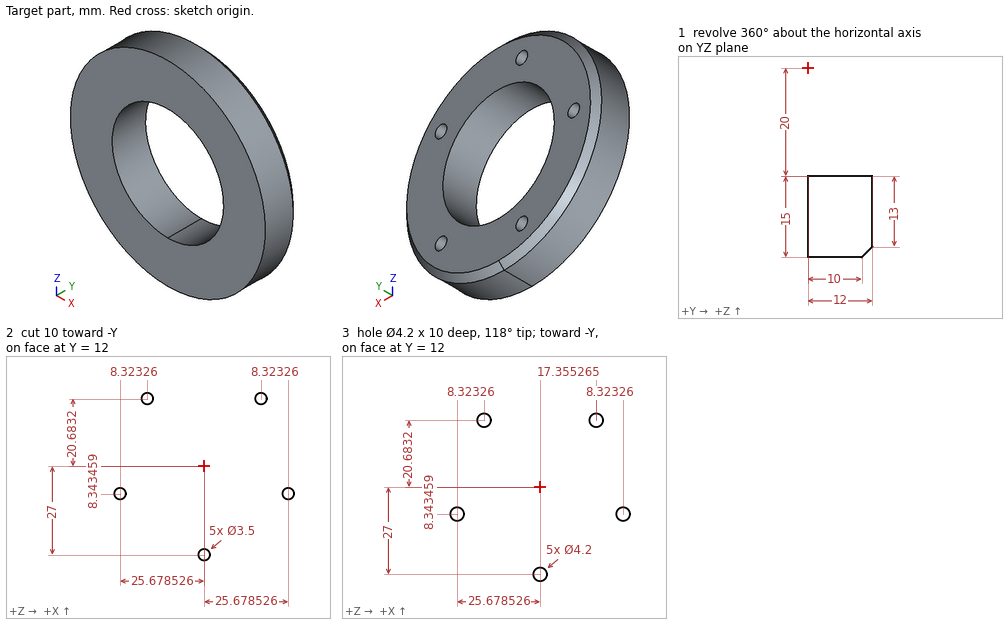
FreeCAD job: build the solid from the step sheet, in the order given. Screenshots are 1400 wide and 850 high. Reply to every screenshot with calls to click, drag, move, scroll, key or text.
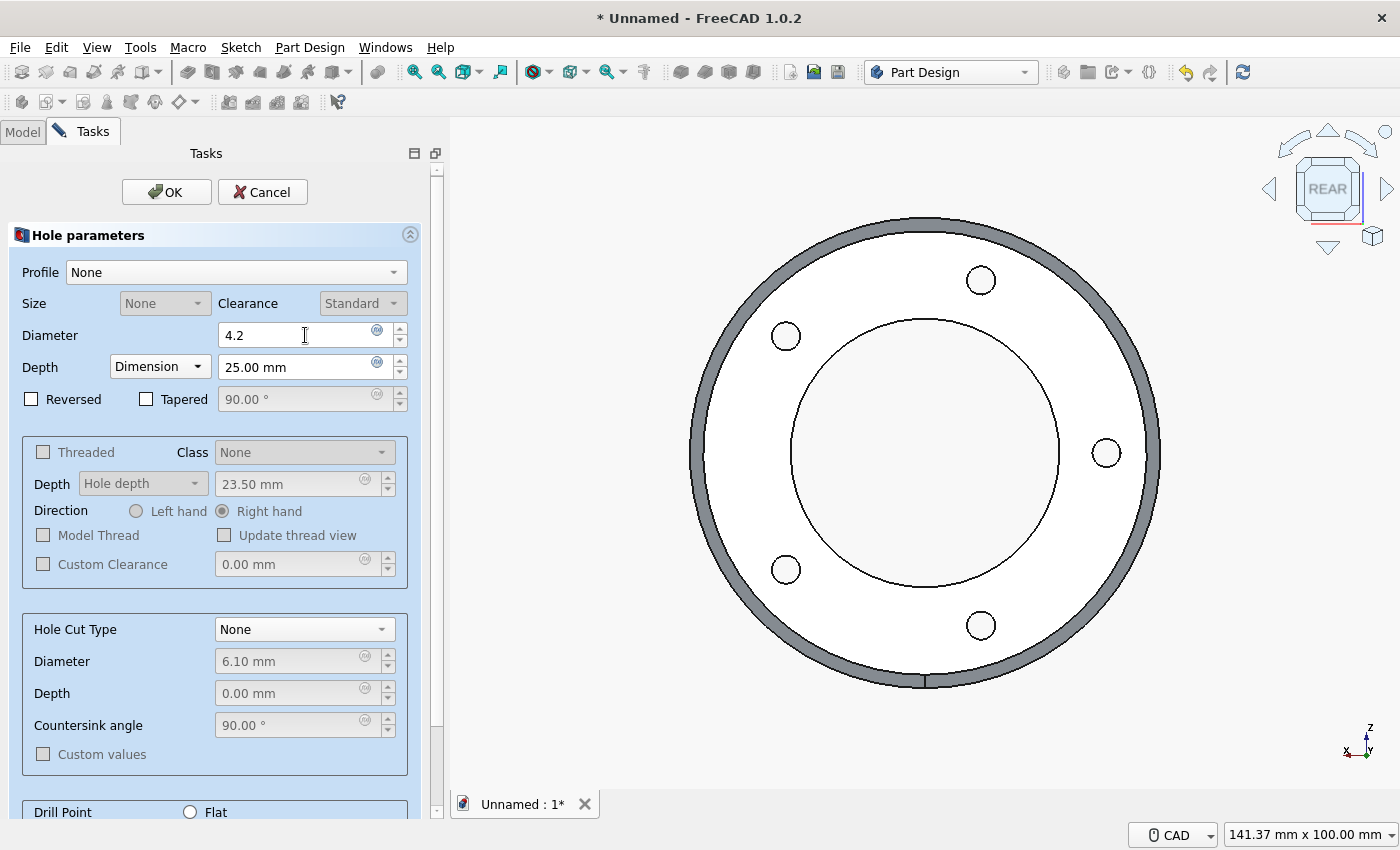
triple_click(305, 367)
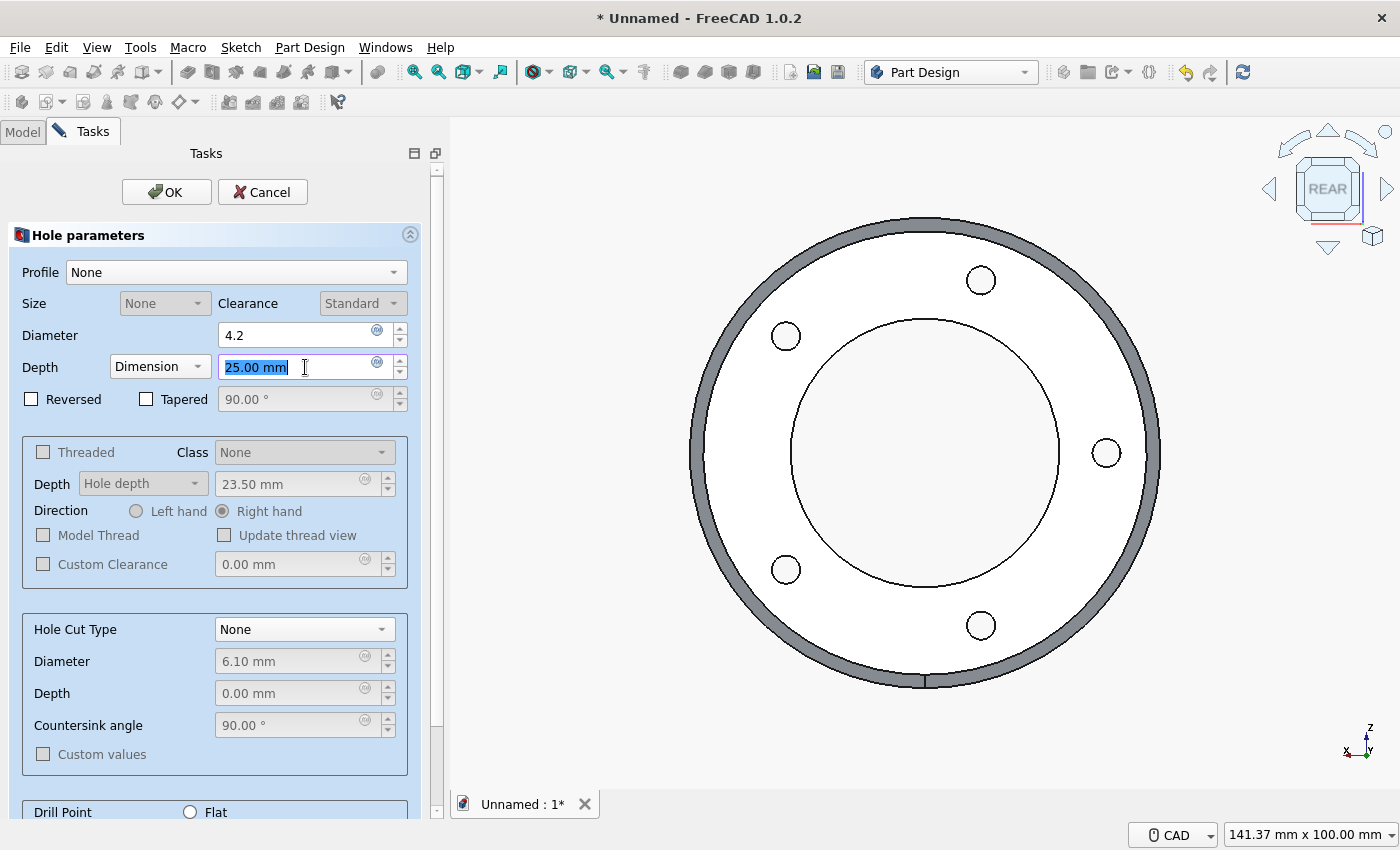
text(10)
key(Tab)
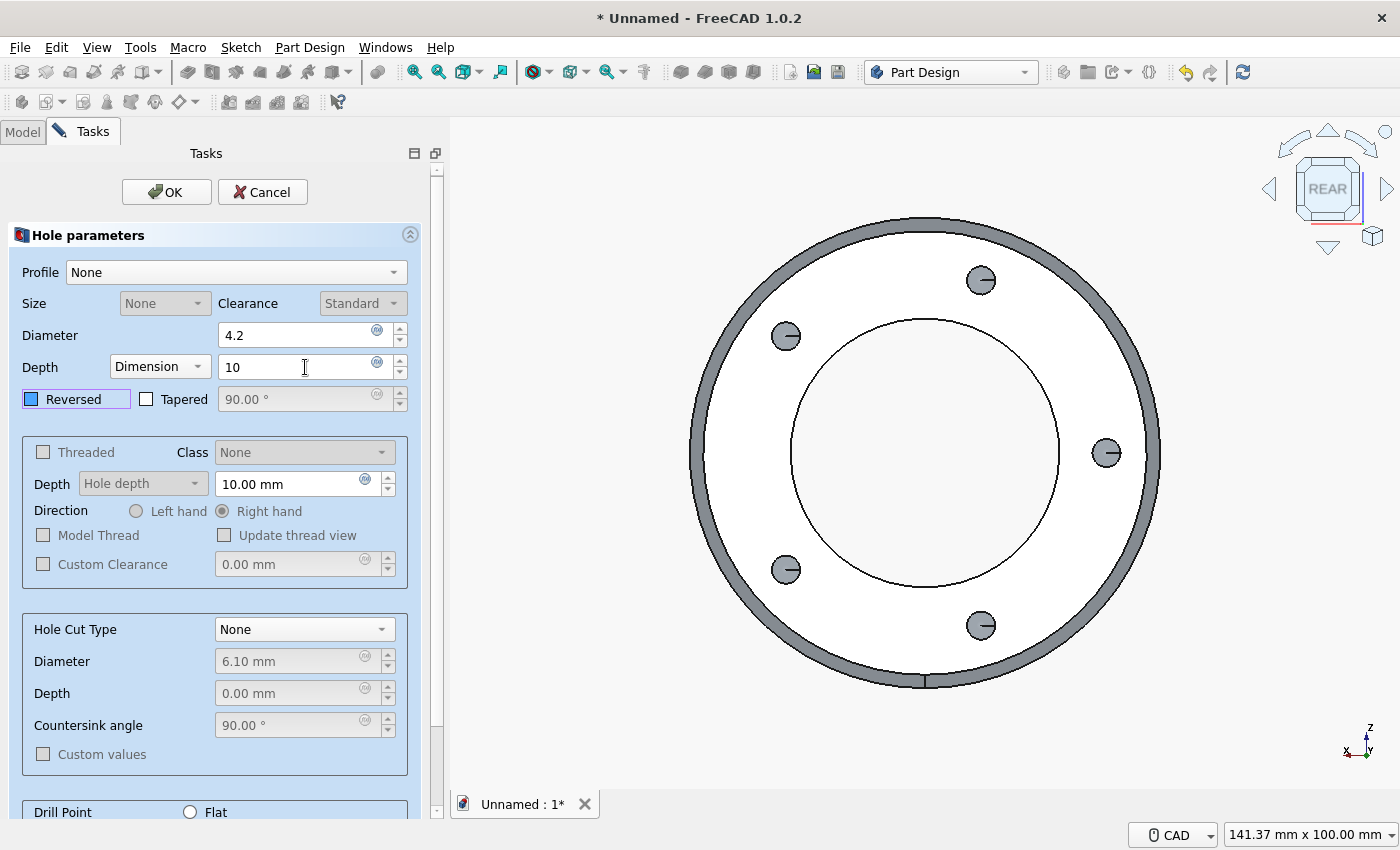
click(167, 192)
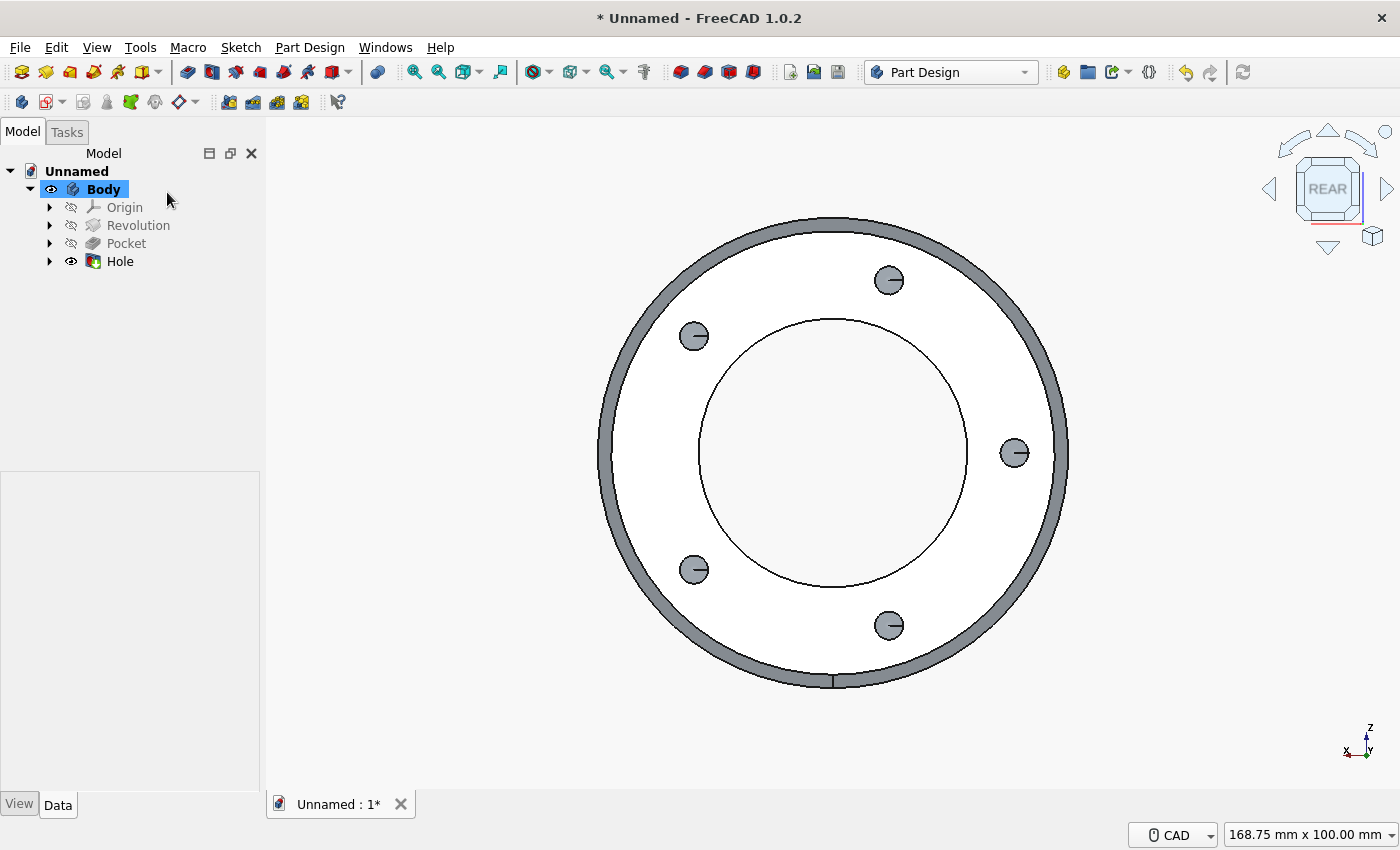
key(0)